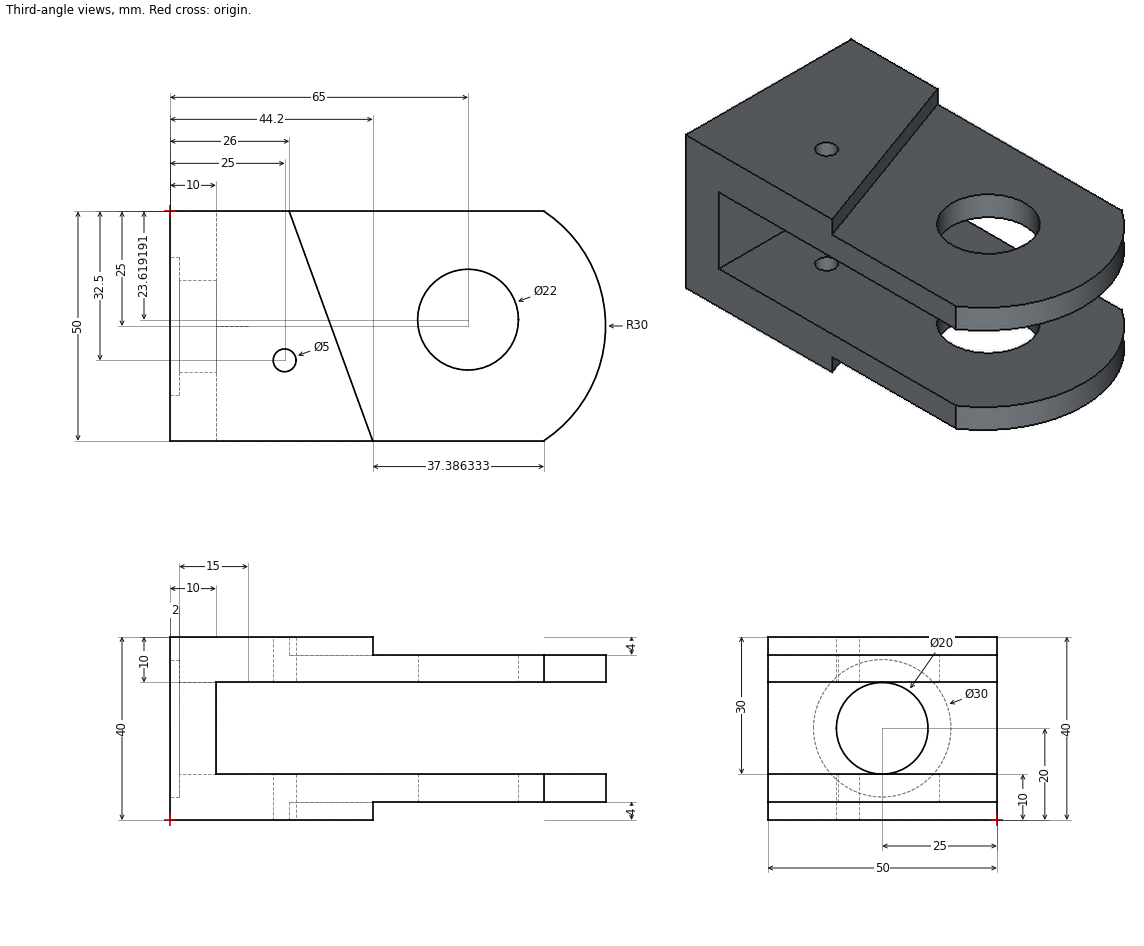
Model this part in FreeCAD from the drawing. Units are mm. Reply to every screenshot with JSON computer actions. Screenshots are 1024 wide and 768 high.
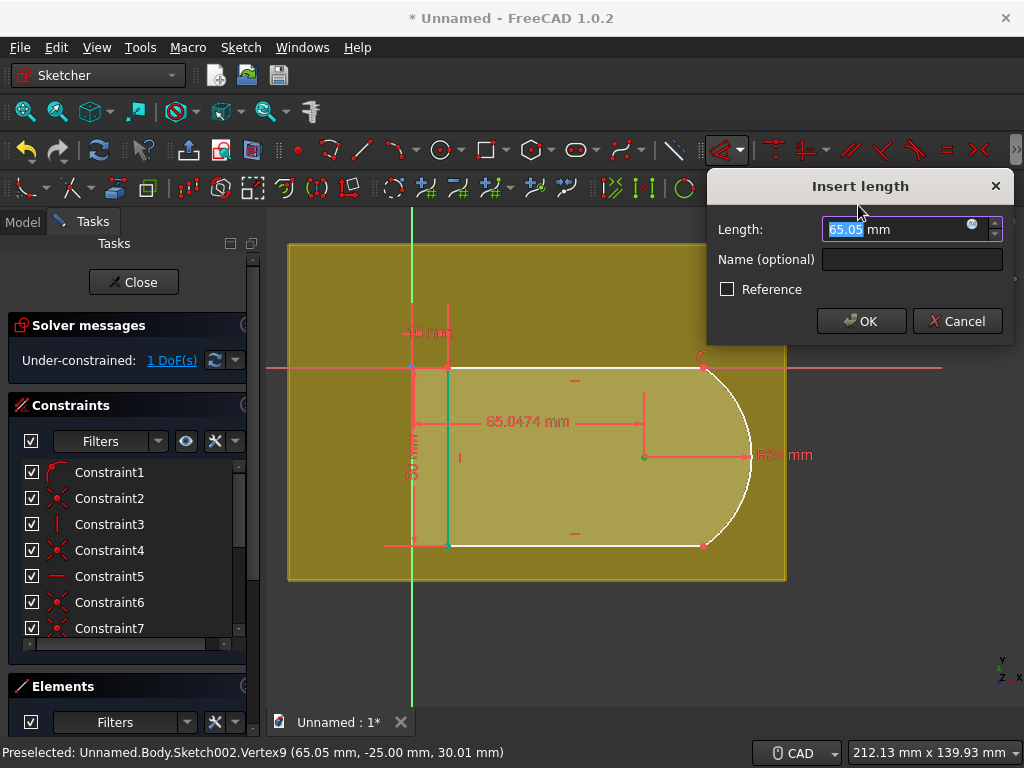
{"action": "type", "text": "65"}
{"action": "key", "text": "Return"}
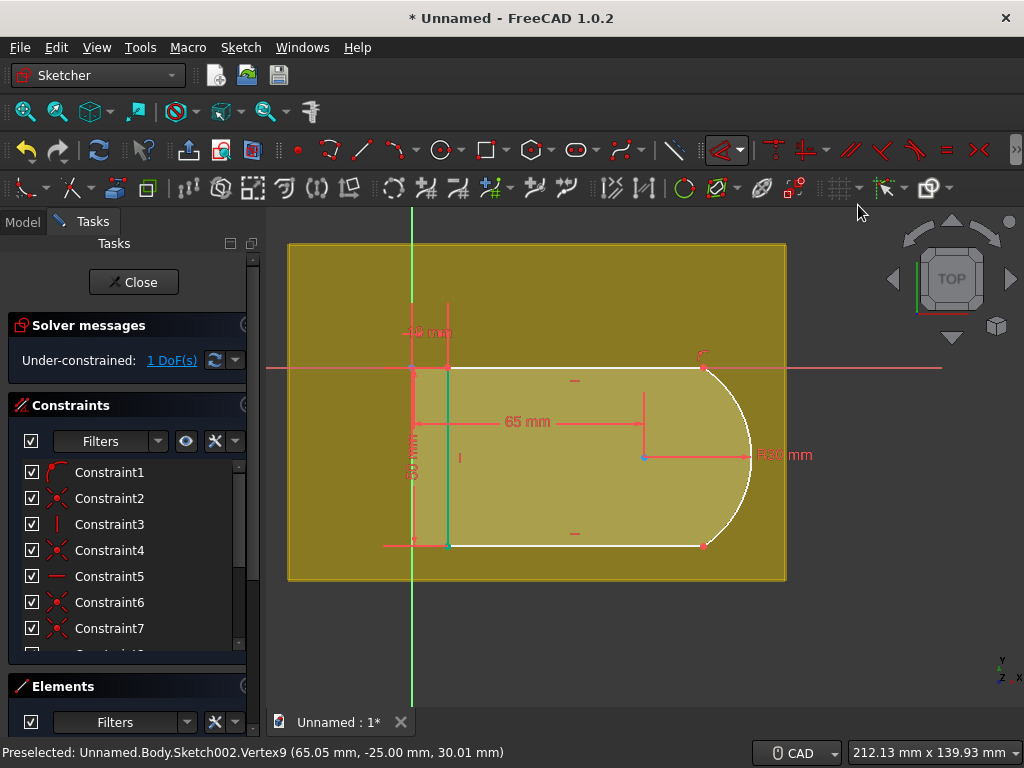
{"action": "left_click", "coordinate": [644, 457]}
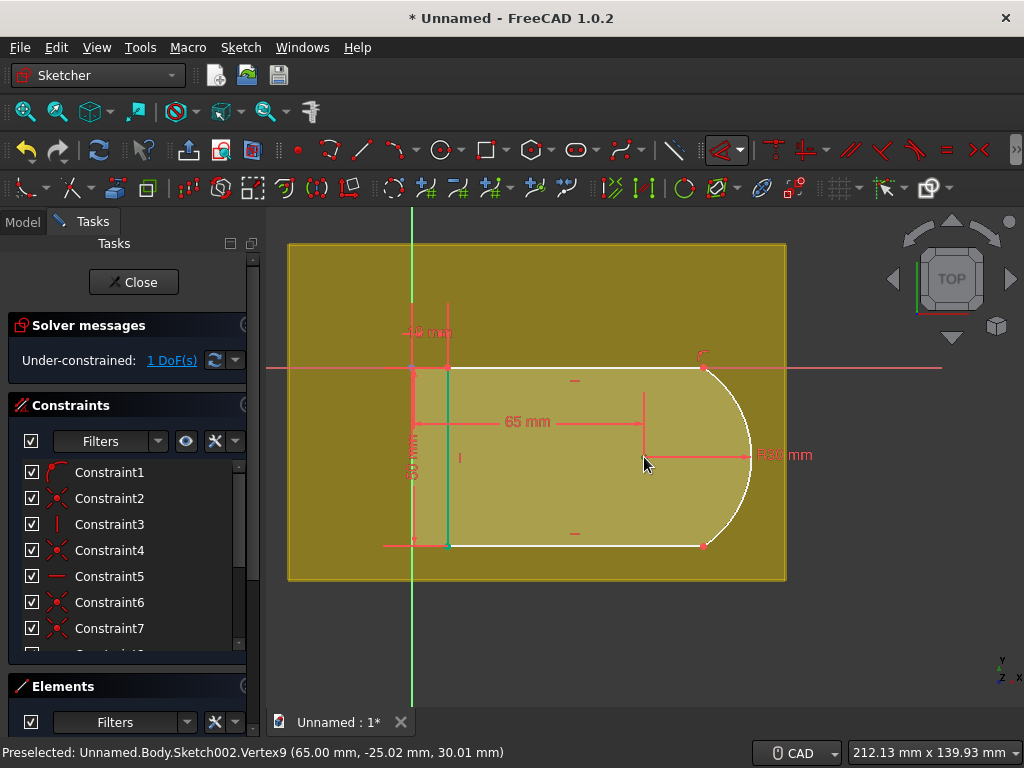
{"action": "key", "text": "i"}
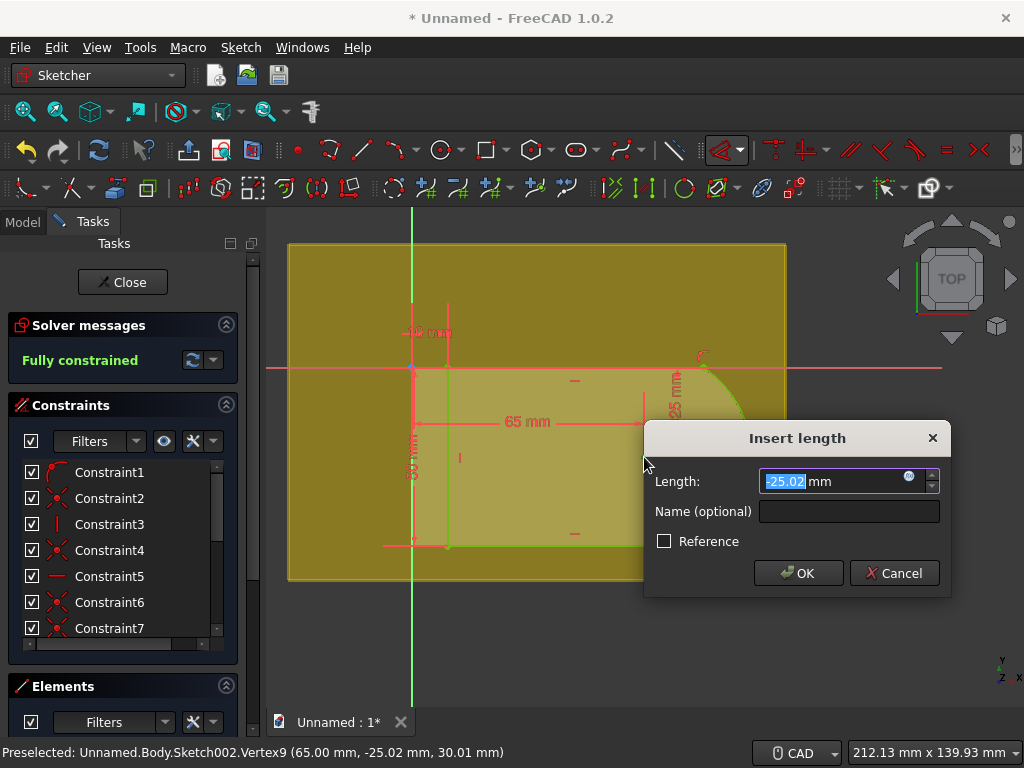
{"action": "type", "text": "-25"}
{"action": "key", "text": "Return"}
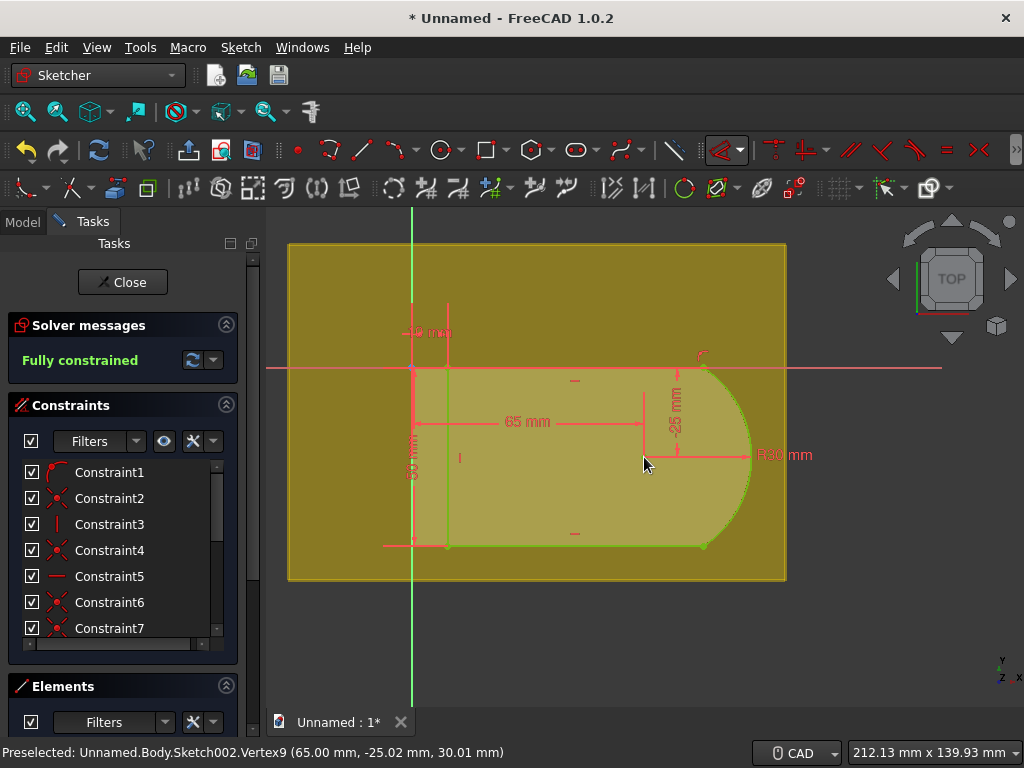
{"action": "left_click", "coordinate": [123, 282]}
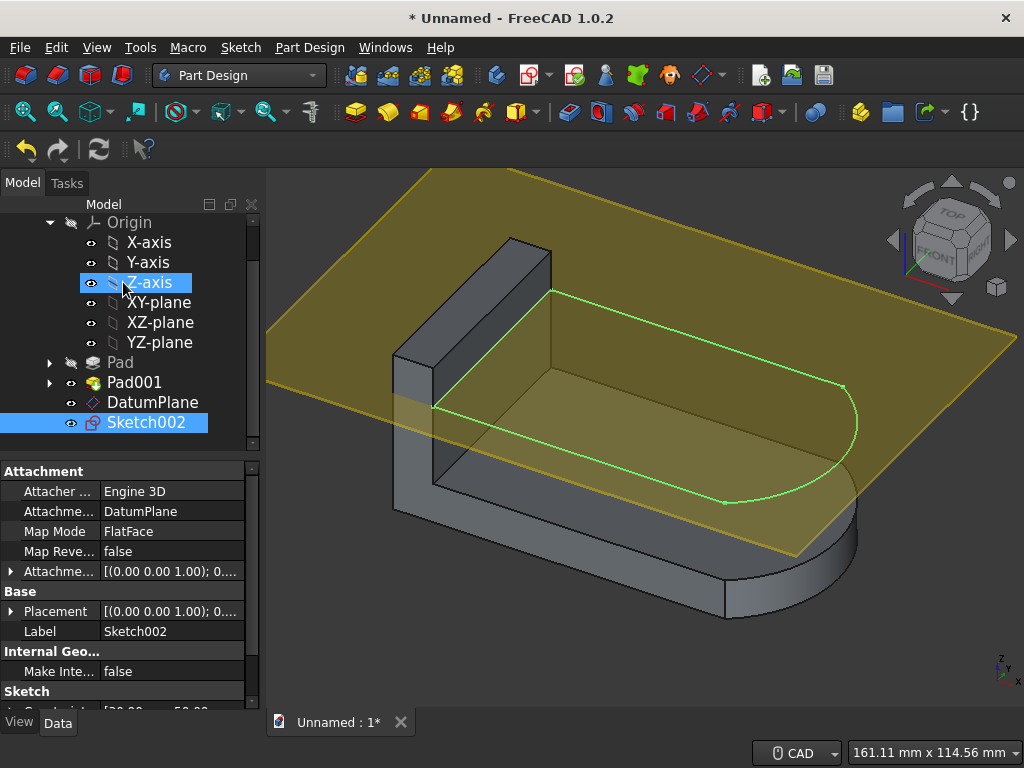
{"action": "left_click", "coordinate": [356, 112]}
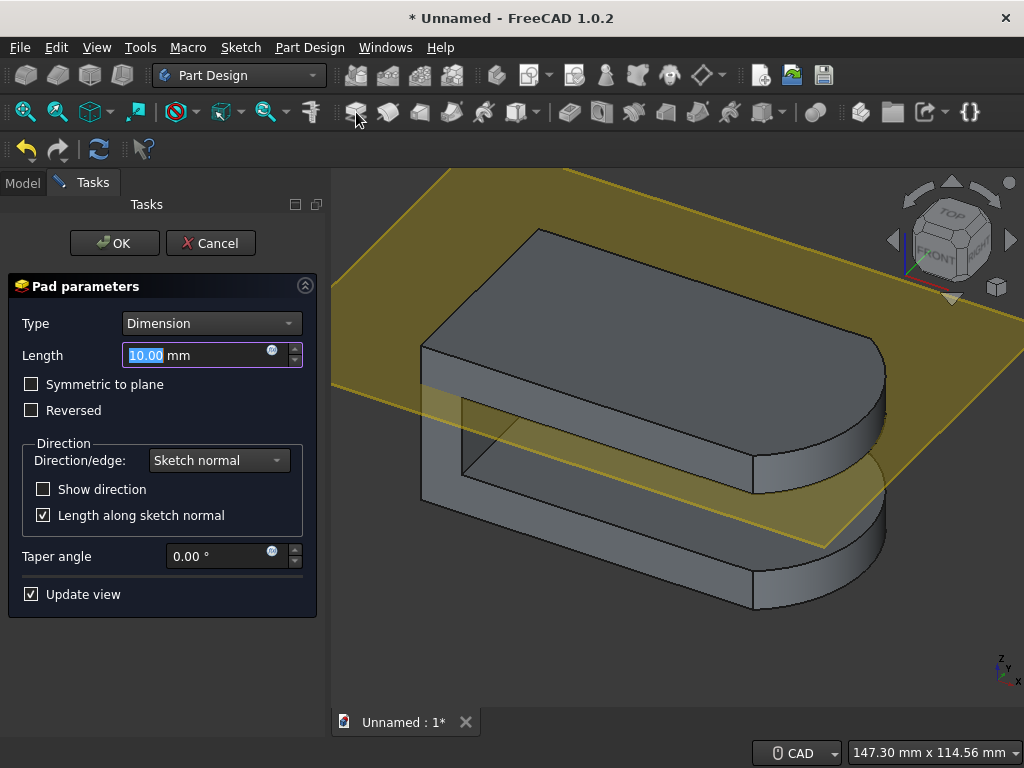
{"action": "type", "text": "10"}
{"action": "key", "text": "Tab"}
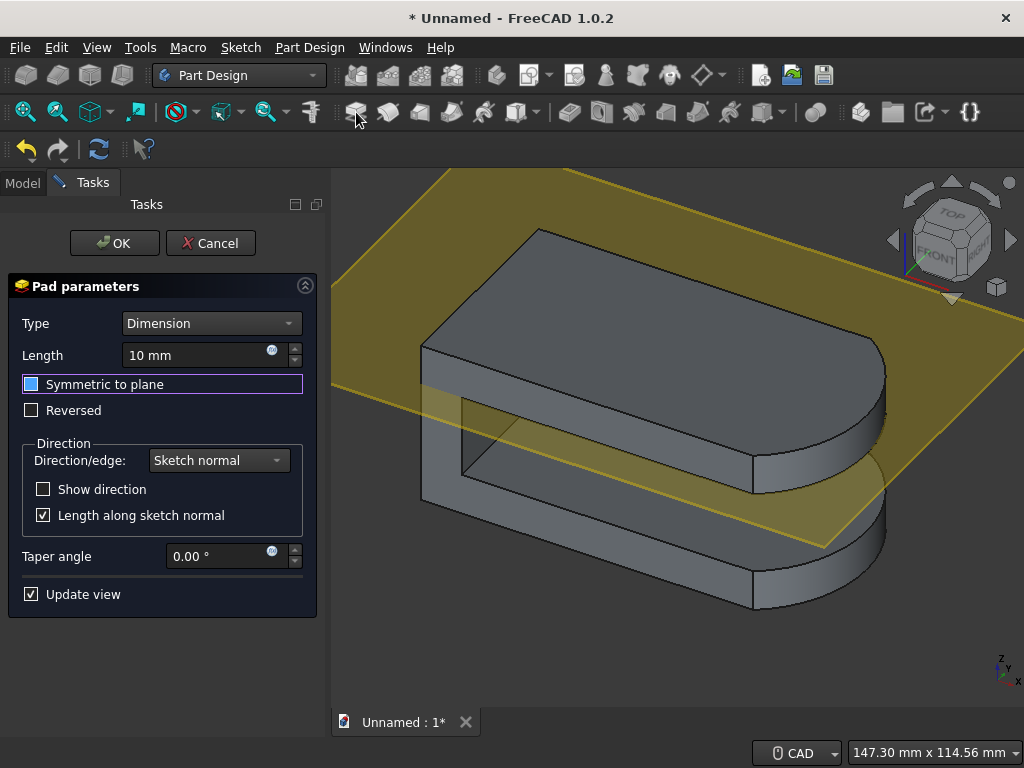
{"action": "left_click", "coordinate": [115, 243]}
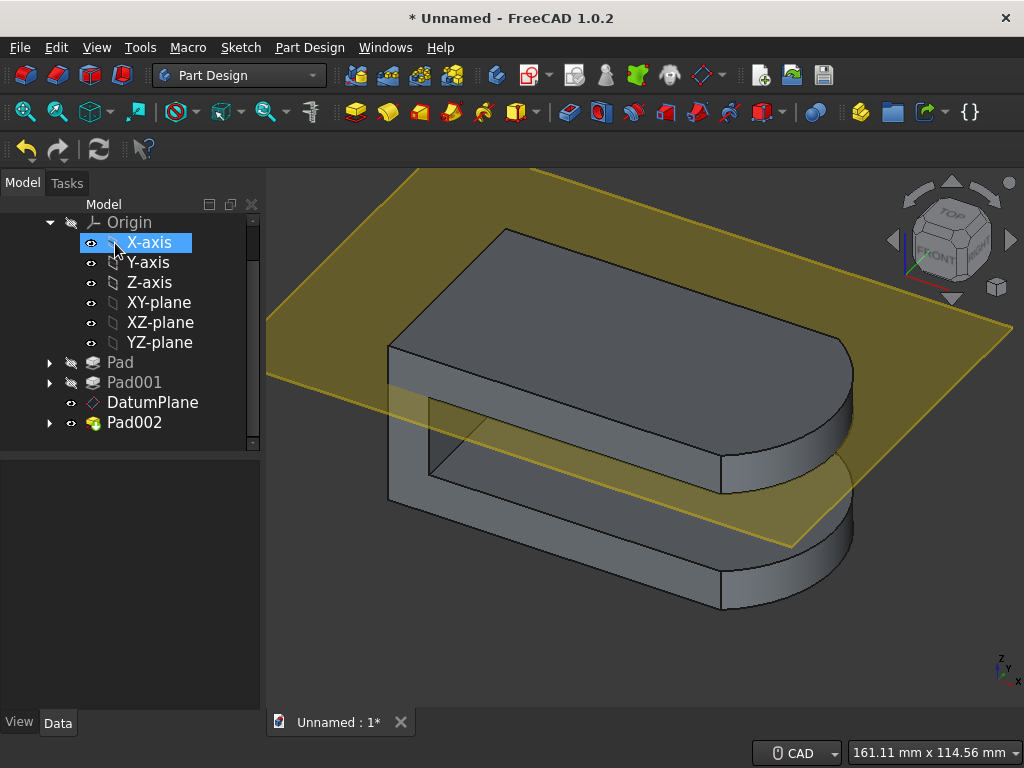
{"action": "left_click", "coordinate": [116, 403]}
{"action": "key", "text": "space"}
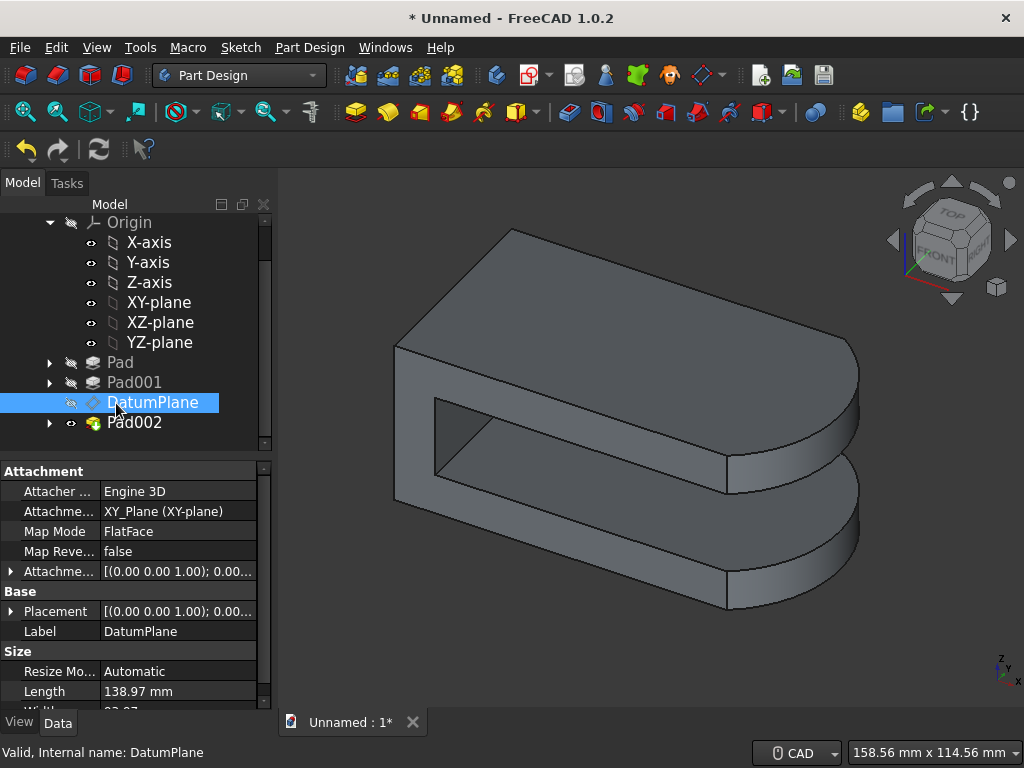
{"action": "left_click", "coordinate": [136, 303]}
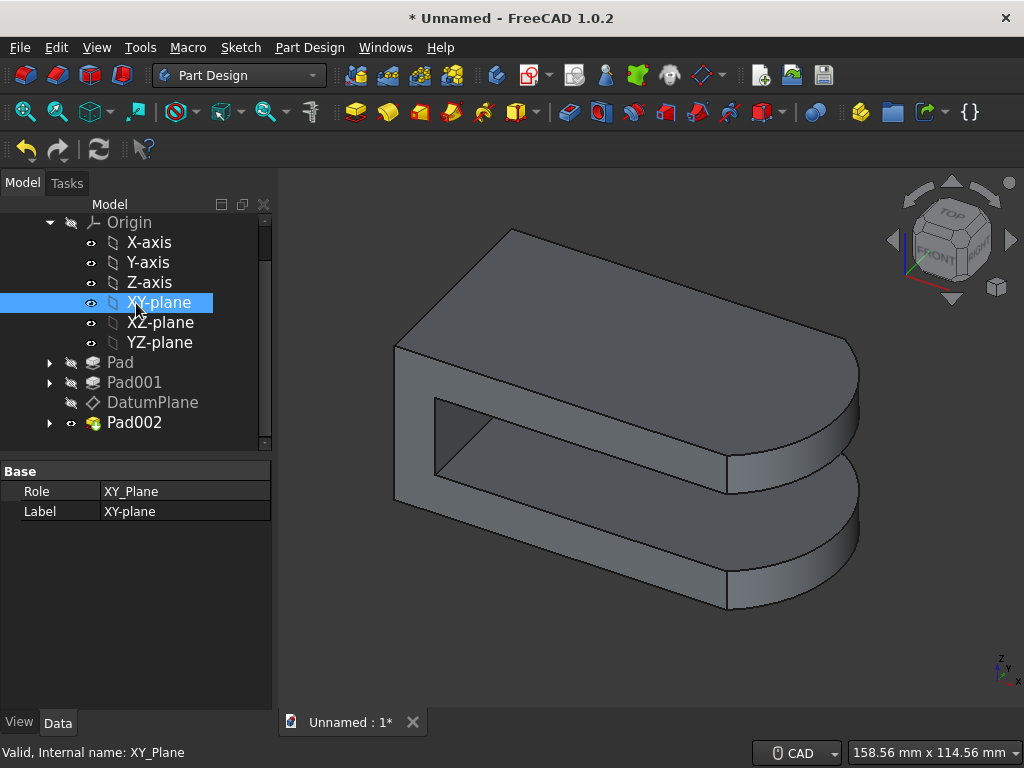
{"action": "left_click", "coordinate": [702, 76]}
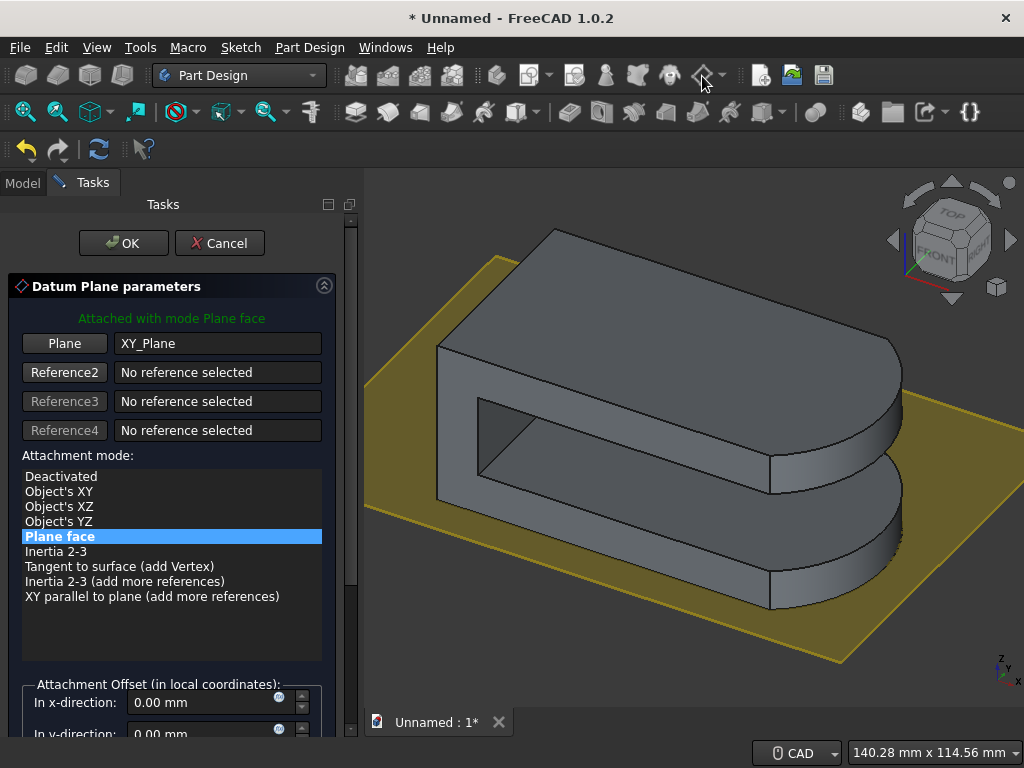
{"action": "scroll", "coordinate": [351, 475], "scroll_direction": "down", "scroll_amount": 2}